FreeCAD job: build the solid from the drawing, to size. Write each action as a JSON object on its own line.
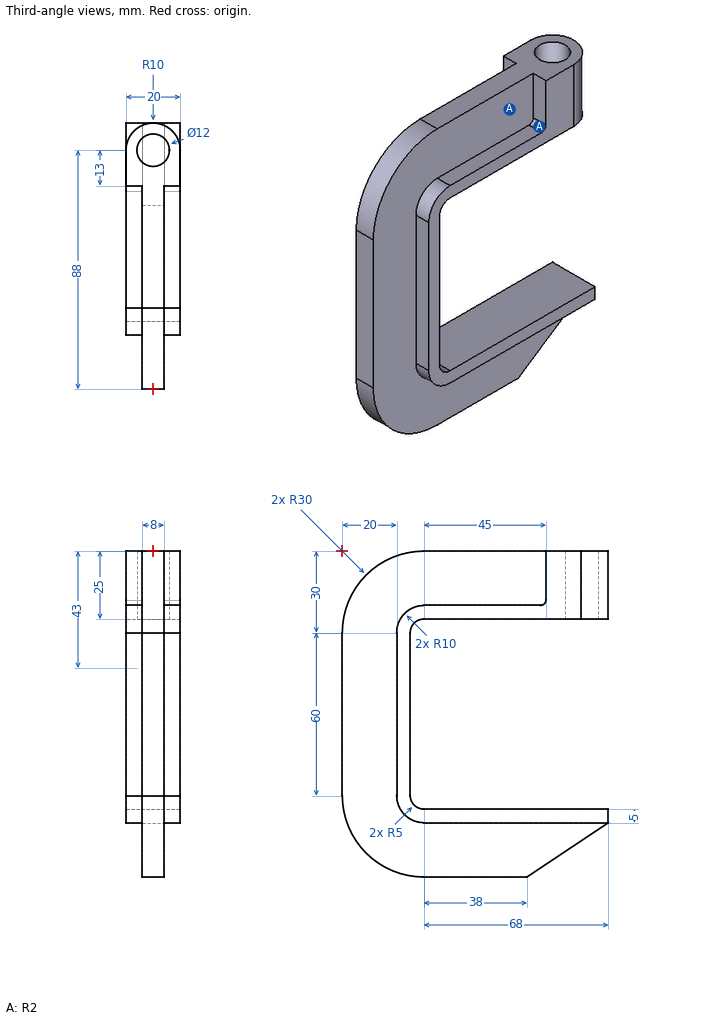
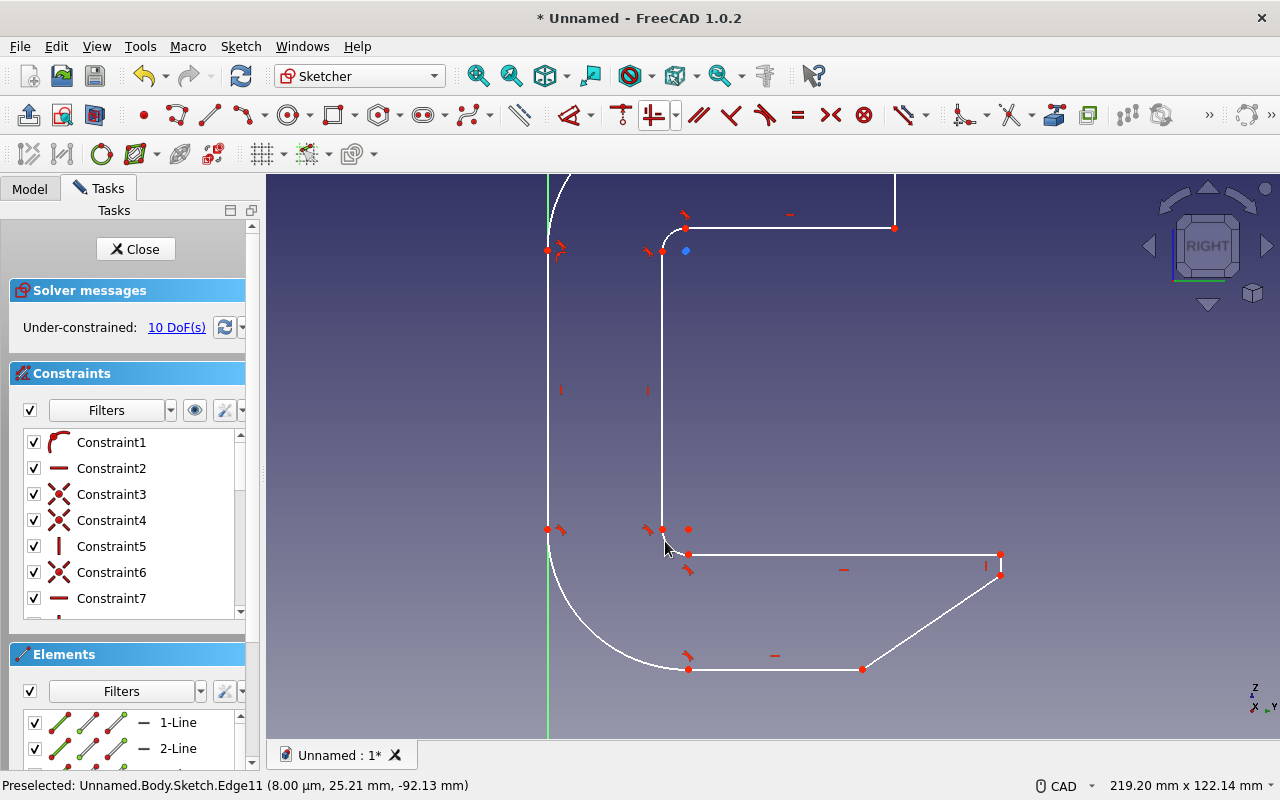
{"action": "scroll", "coordinate": [675, 231], "scroll_direction": "up", "scroll_amount": 2}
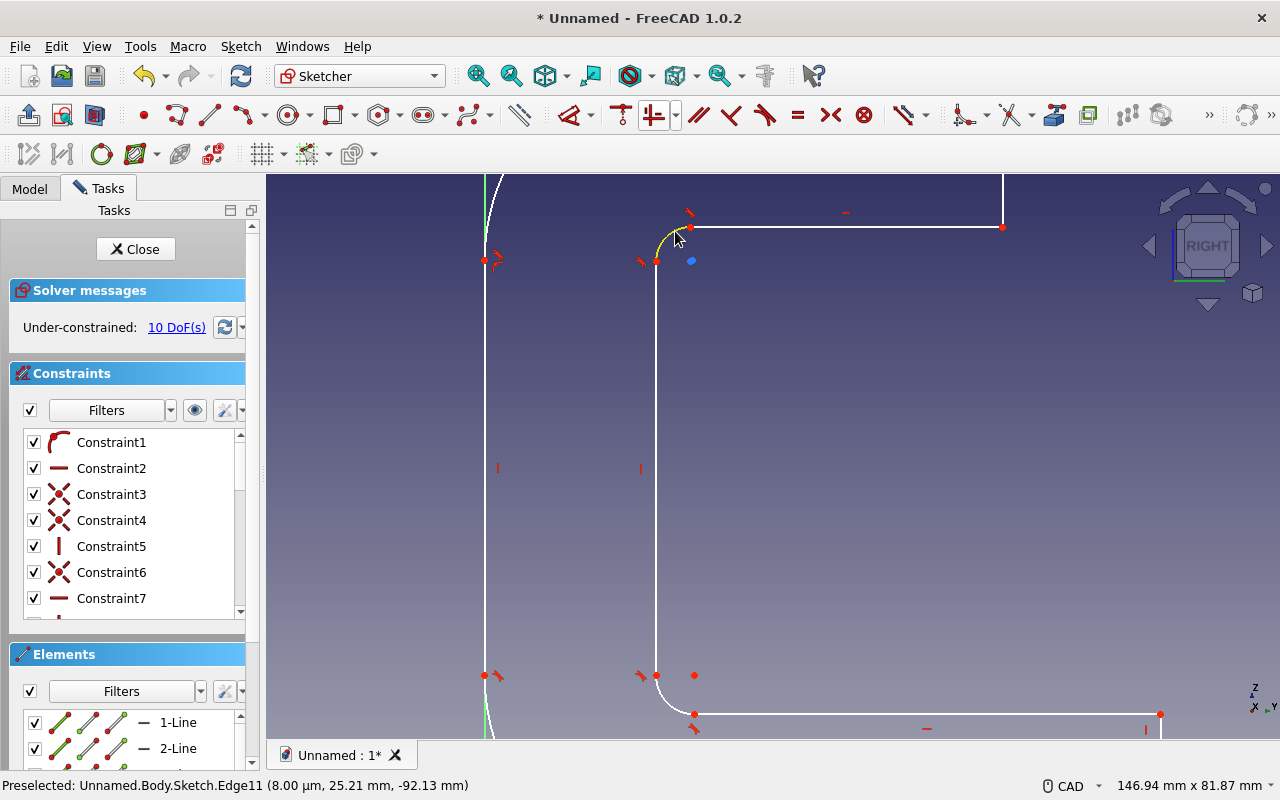
{"action": "left_click", "coordinate": [675, 231]}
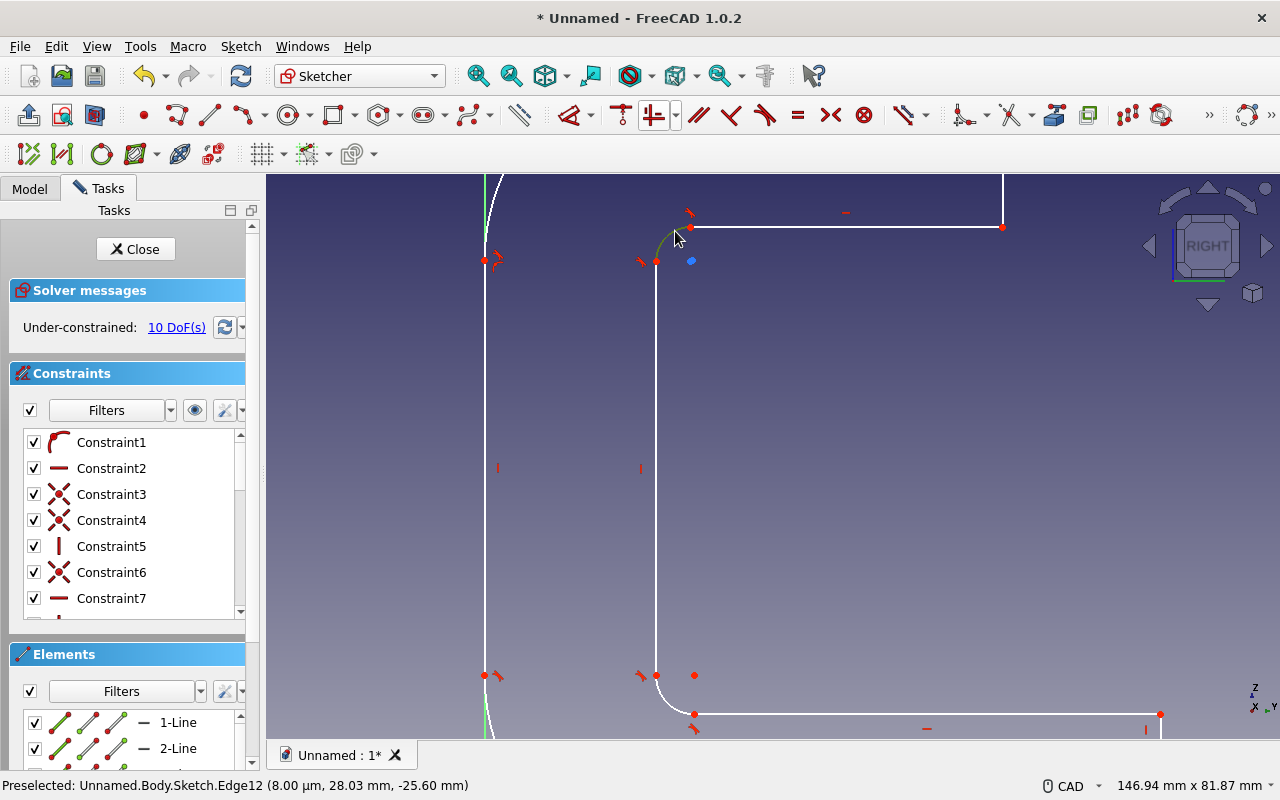
{"action": "scroll", "coordinate": [608, 448], "scroll_direction": "down", "scroll_amount": 4}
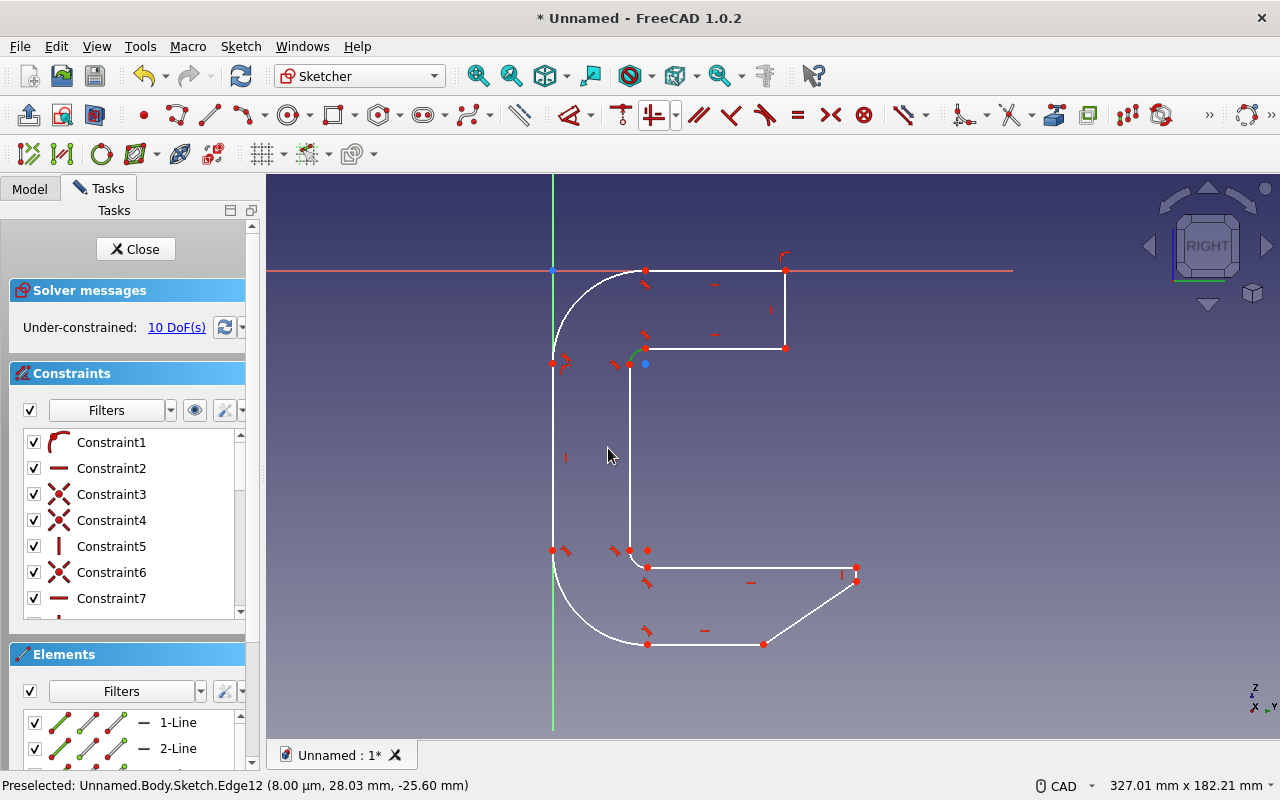
{"action": "scroll", "coordinate": [604, 281], "scroll_direction": "up", "scroll_amount": 2}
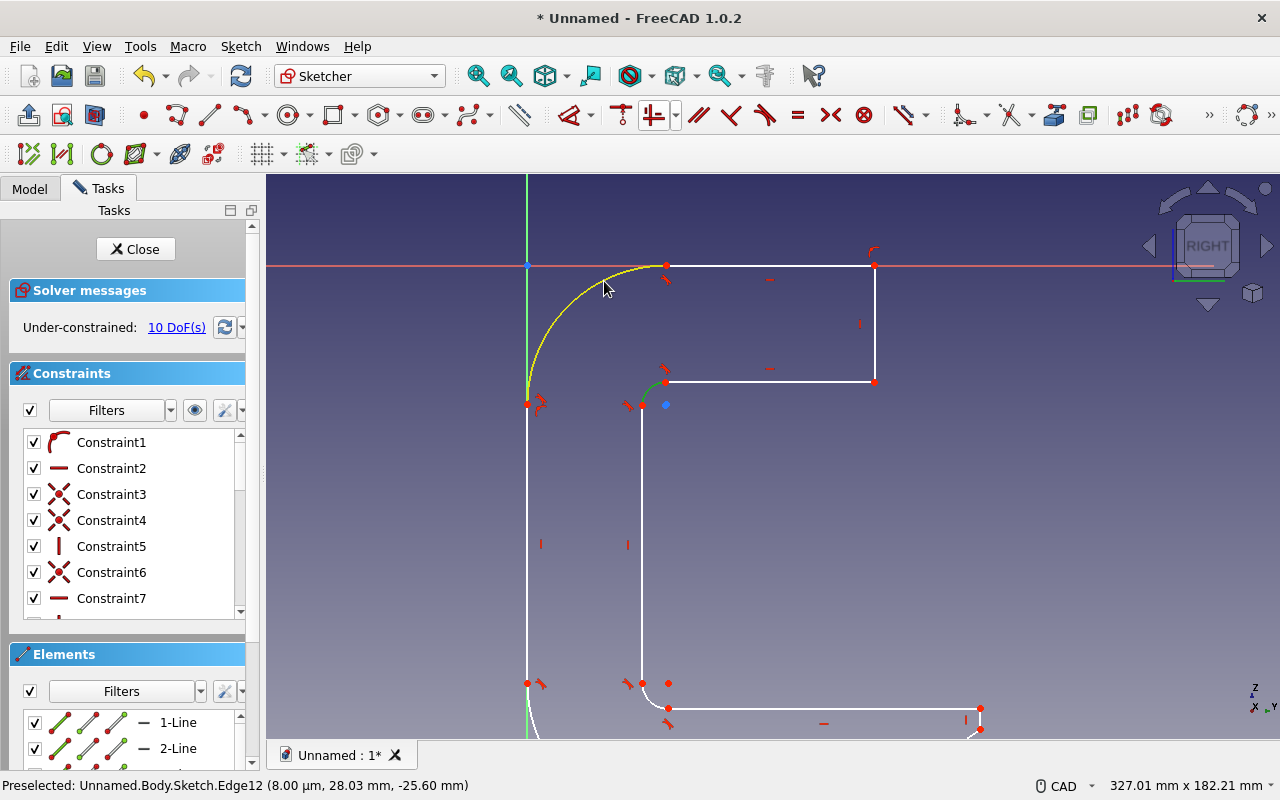
{"action": "left_click", "coordinate": [603, 281]}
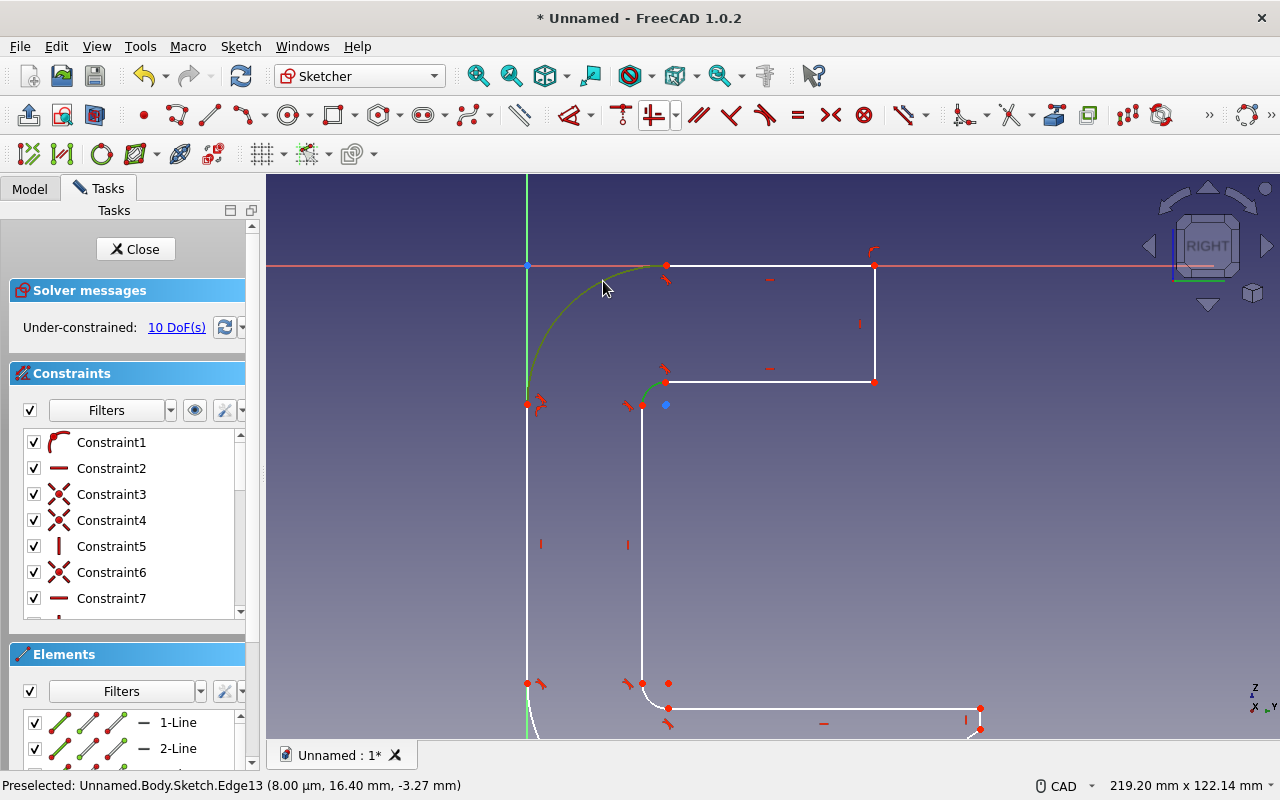
{"action": "left_click", "coordinate": [621, 116]}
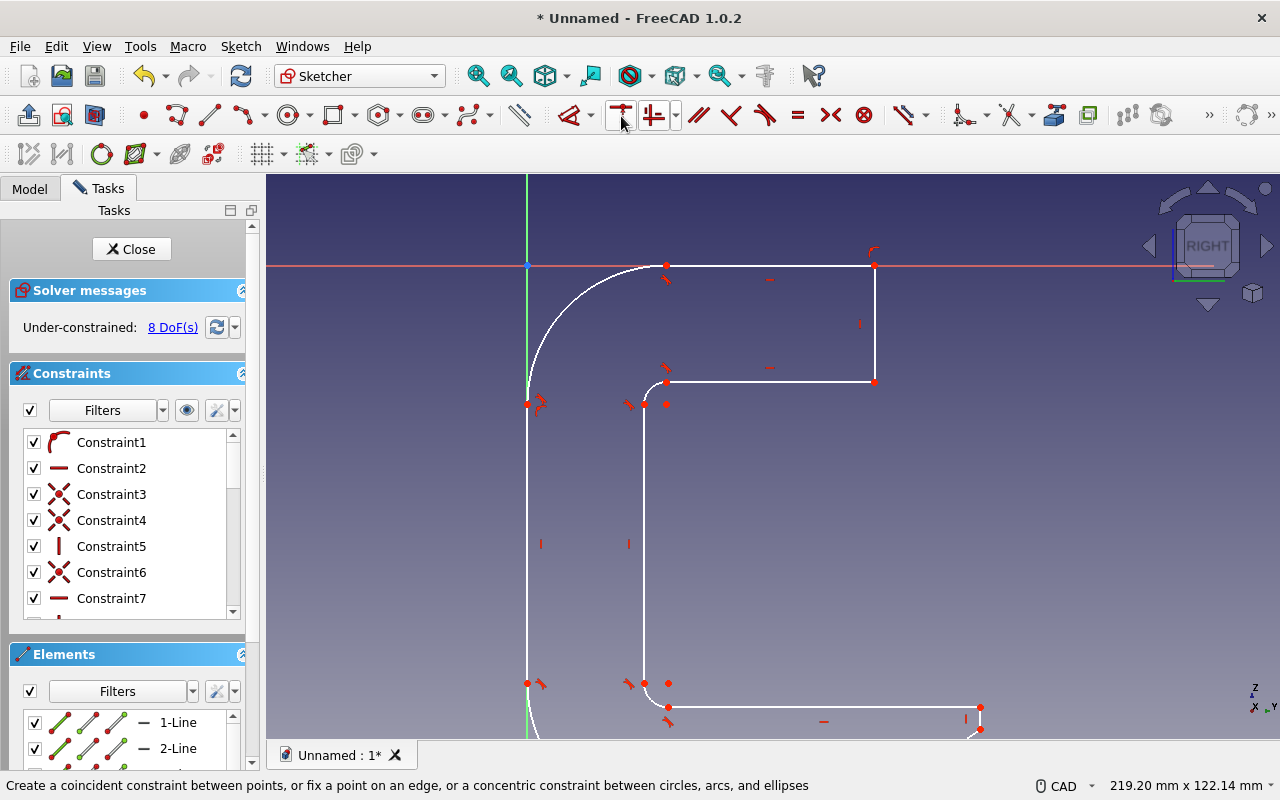
{"action": "scroll", "coordinate": [647, 694], "scroll_direction": "up", "scroll_amount": 2}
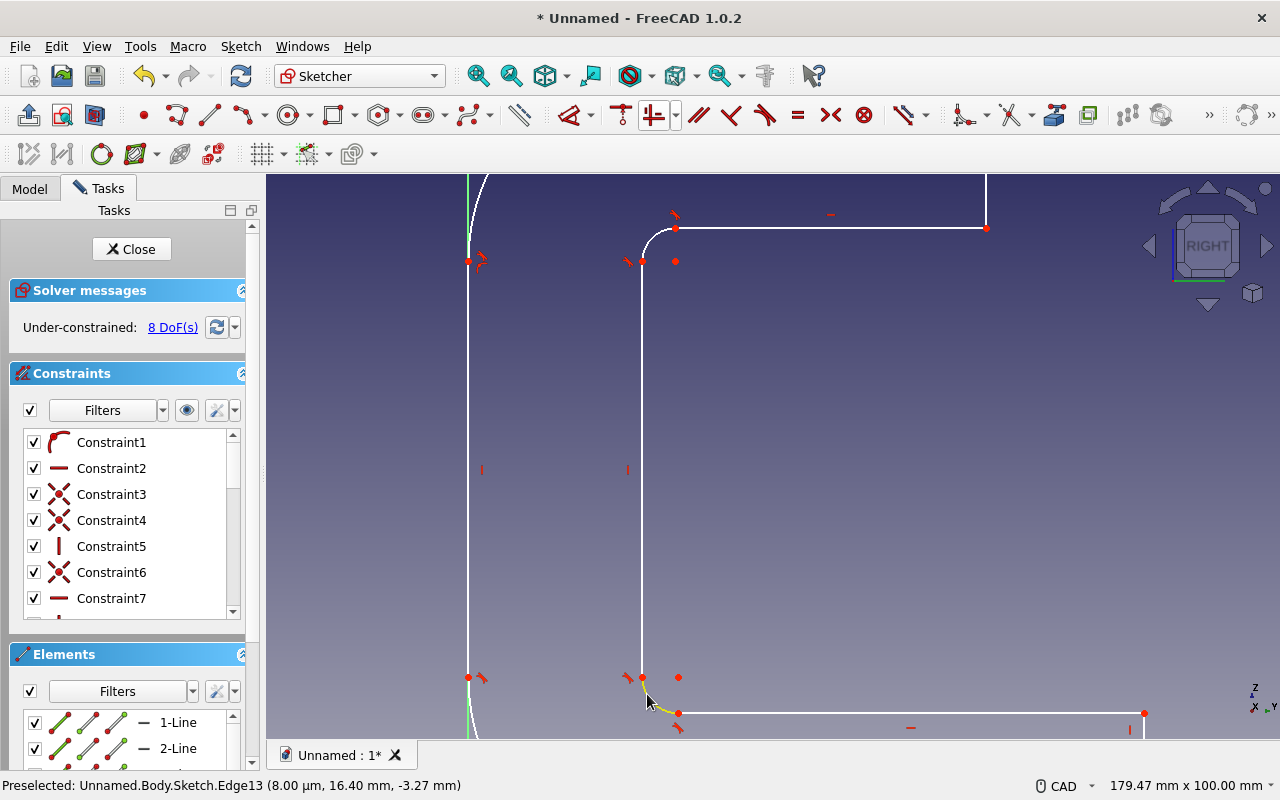
{"action": "left_click", "coordinate": [646, 694]}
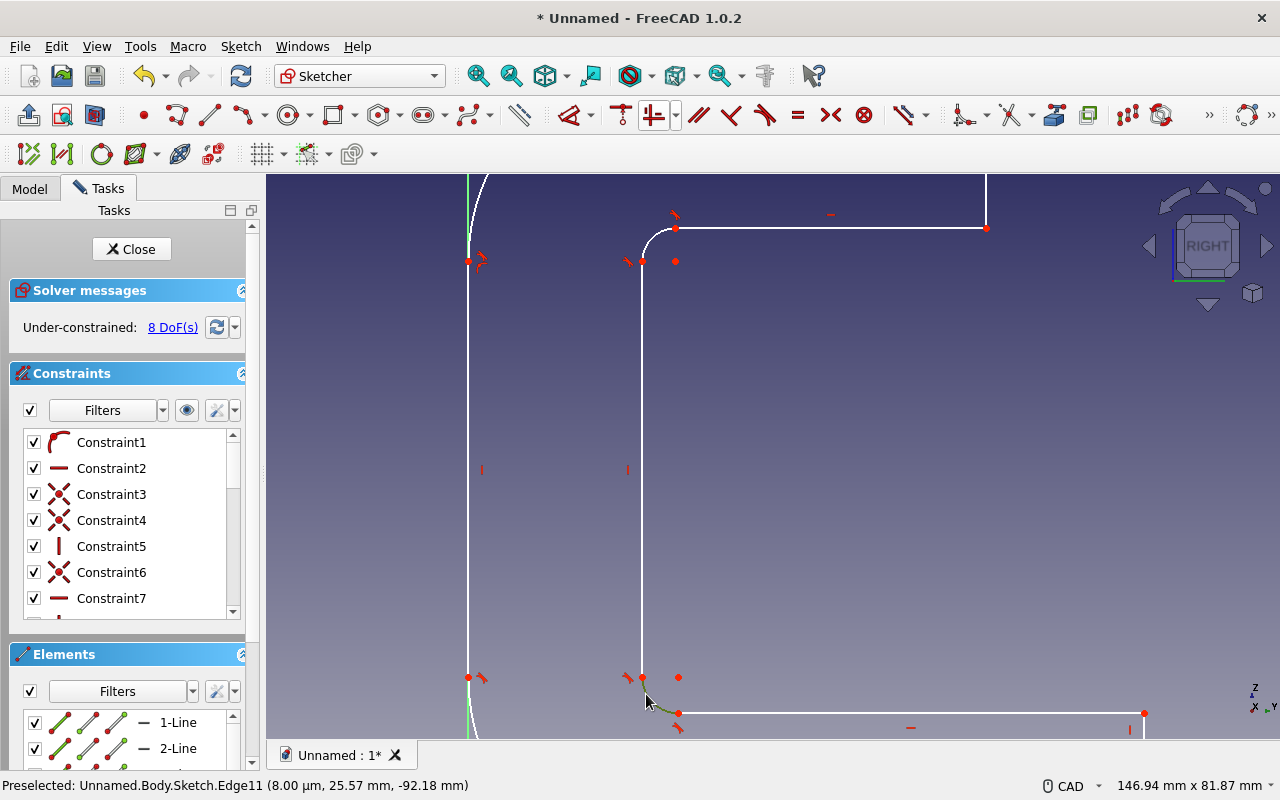
{"action": "left_click", "coordinate": [661, 232]}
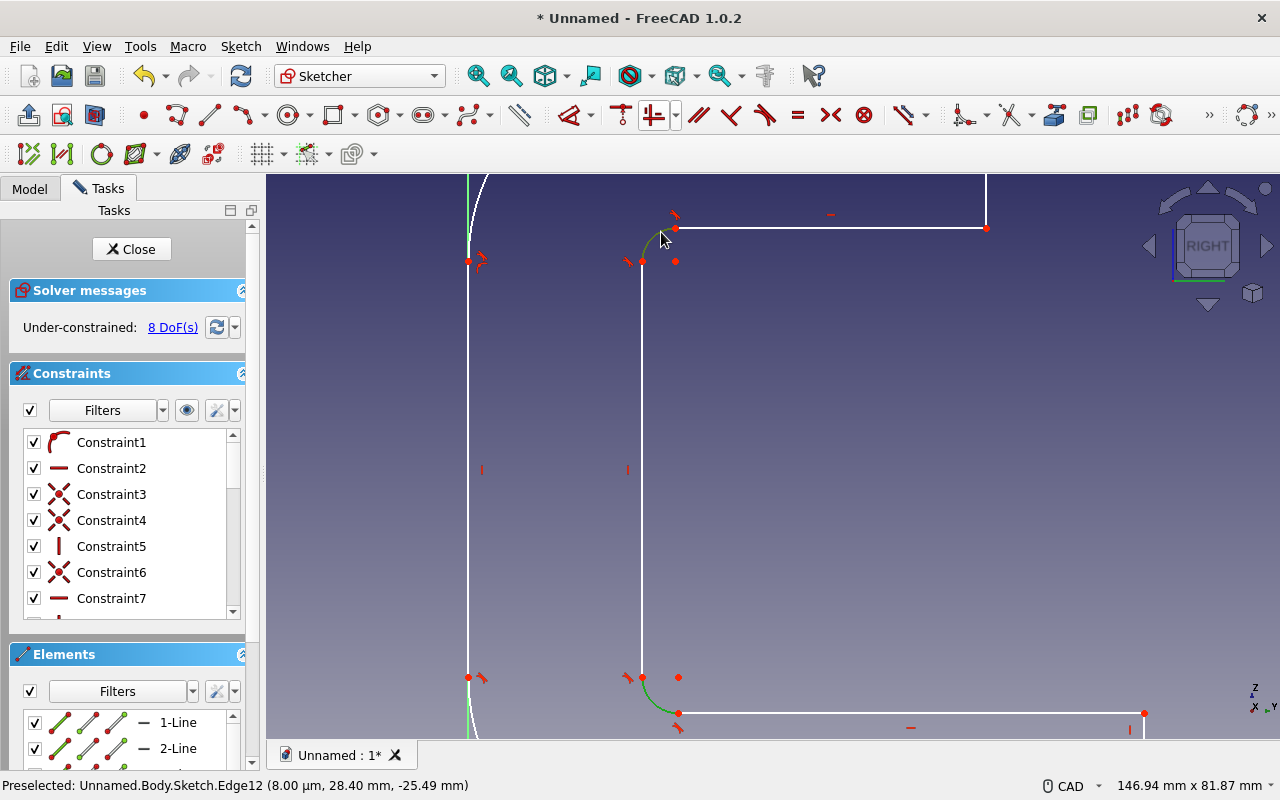
{"action": "key", "text": "e"}